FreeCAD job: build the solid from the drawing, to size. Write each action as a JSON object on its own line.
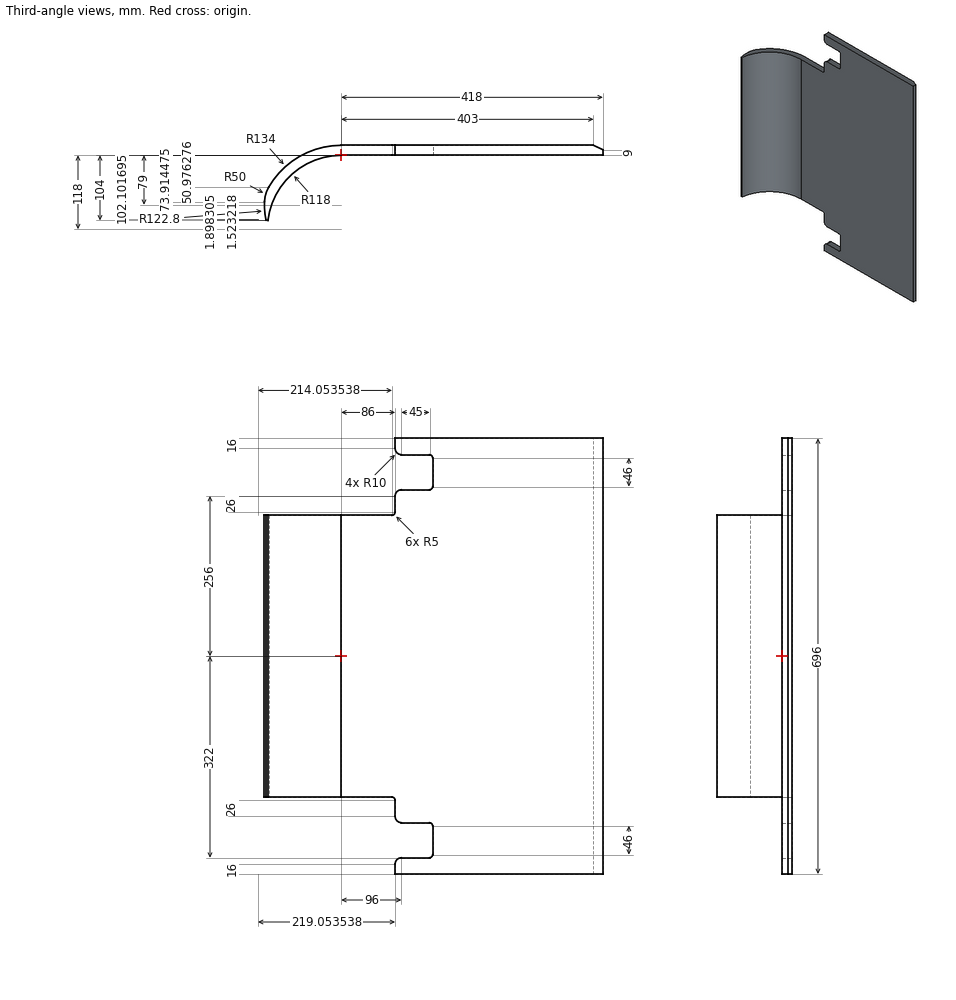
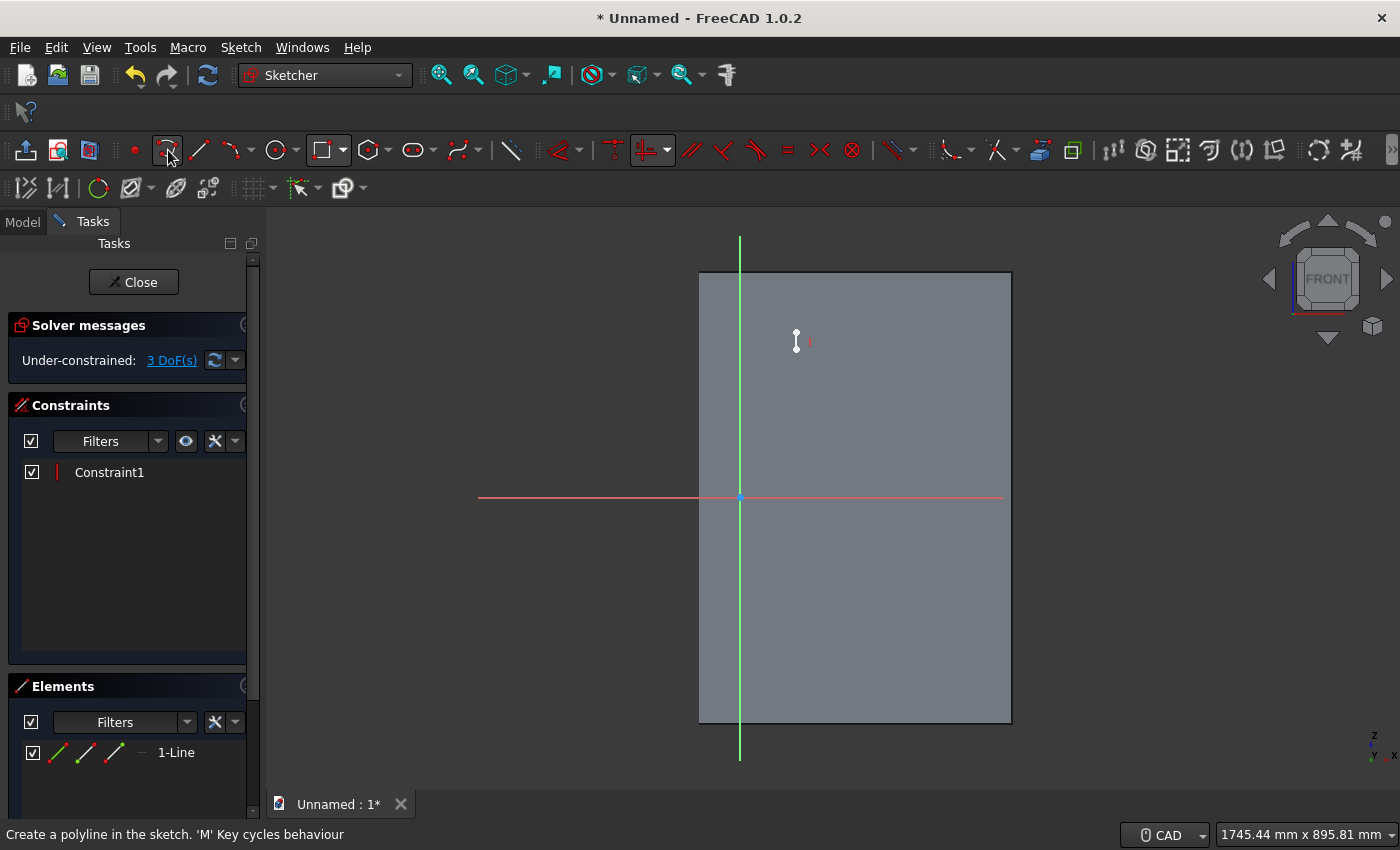
{"action": "scroll", "coordinate": [793, 352], "scroll_direction": "up", "scroll_amount": 7}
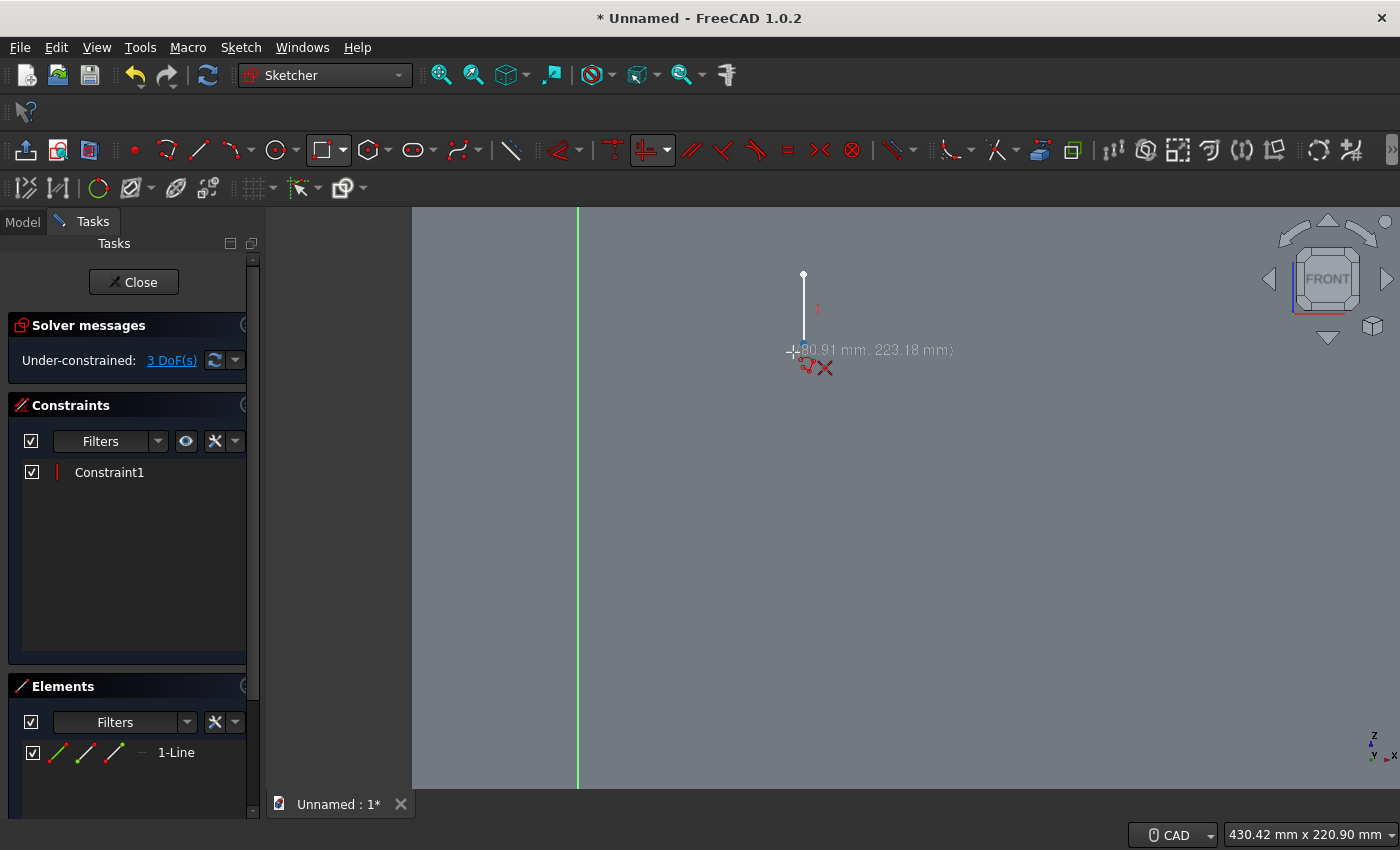
{"action": "left_click", "coordinate": [792, 351]}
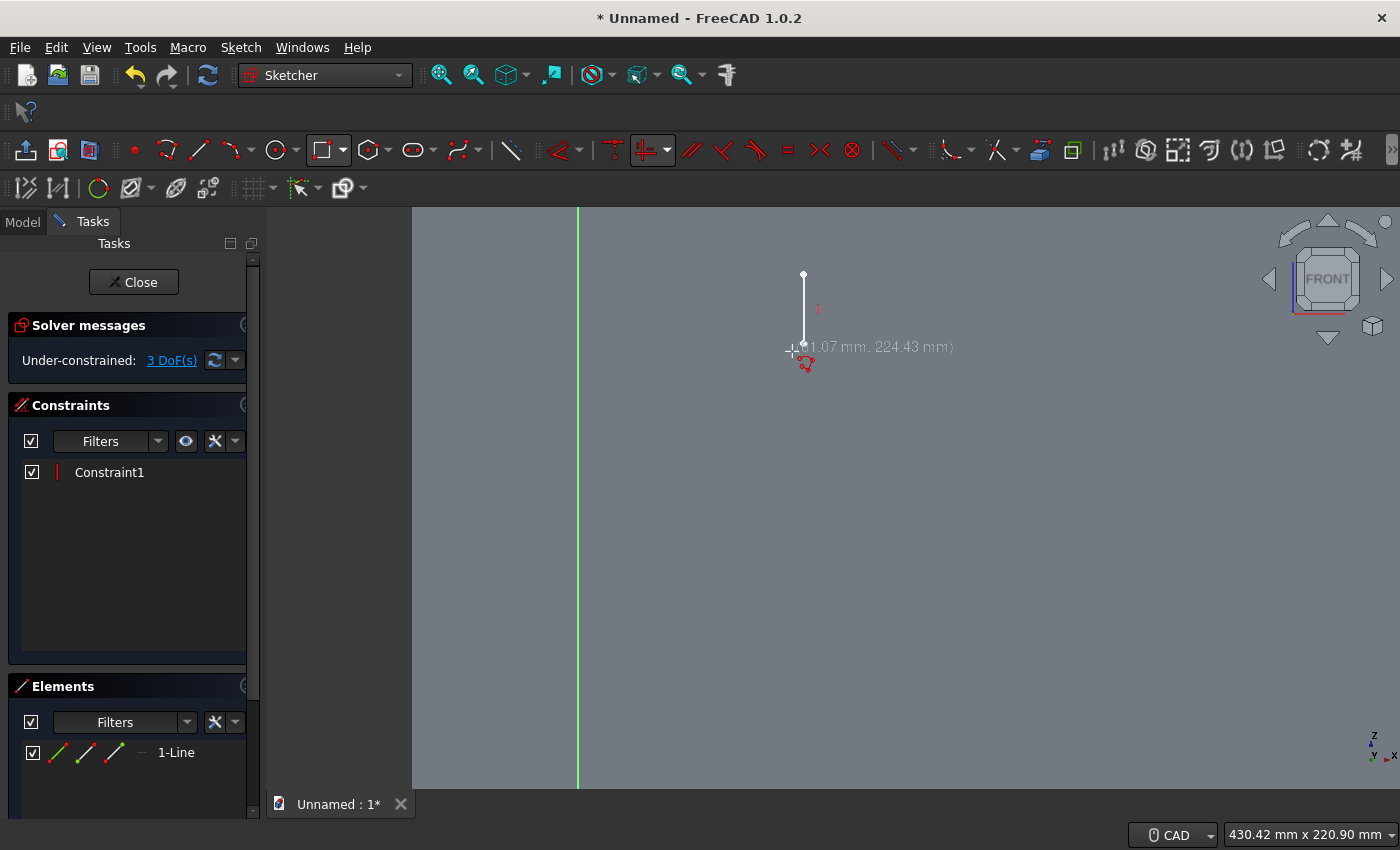
{"action": "scroll", "coordinate": [807, 385], "scroll_direction": "down", "scroll_amount": 8}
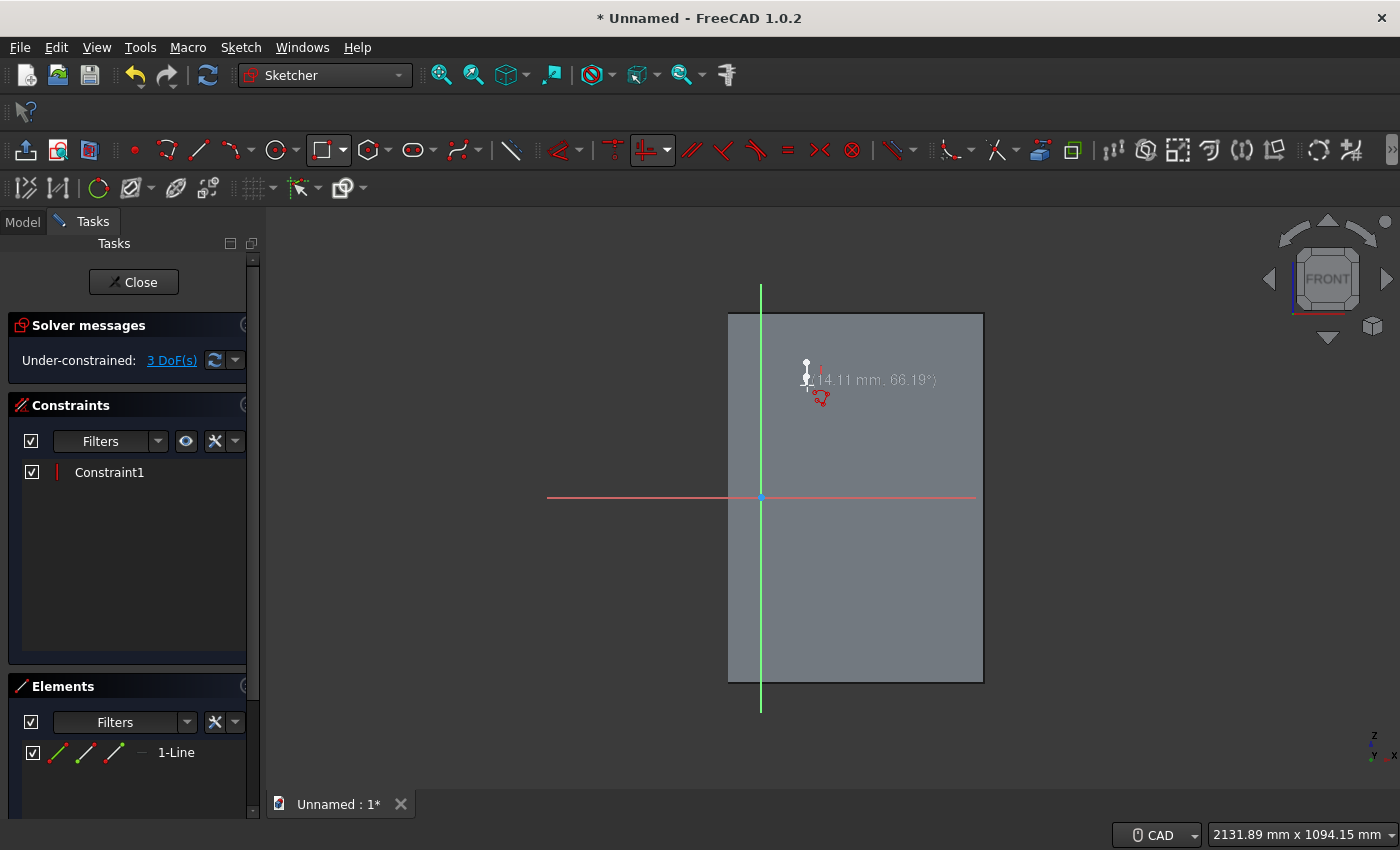
{"action": "left_click", "coordinate": [690, 378]}
{"action": "left_click", "coordinate": [690, 313]}
{"action": "left_click", "coordinate": [807, 313]}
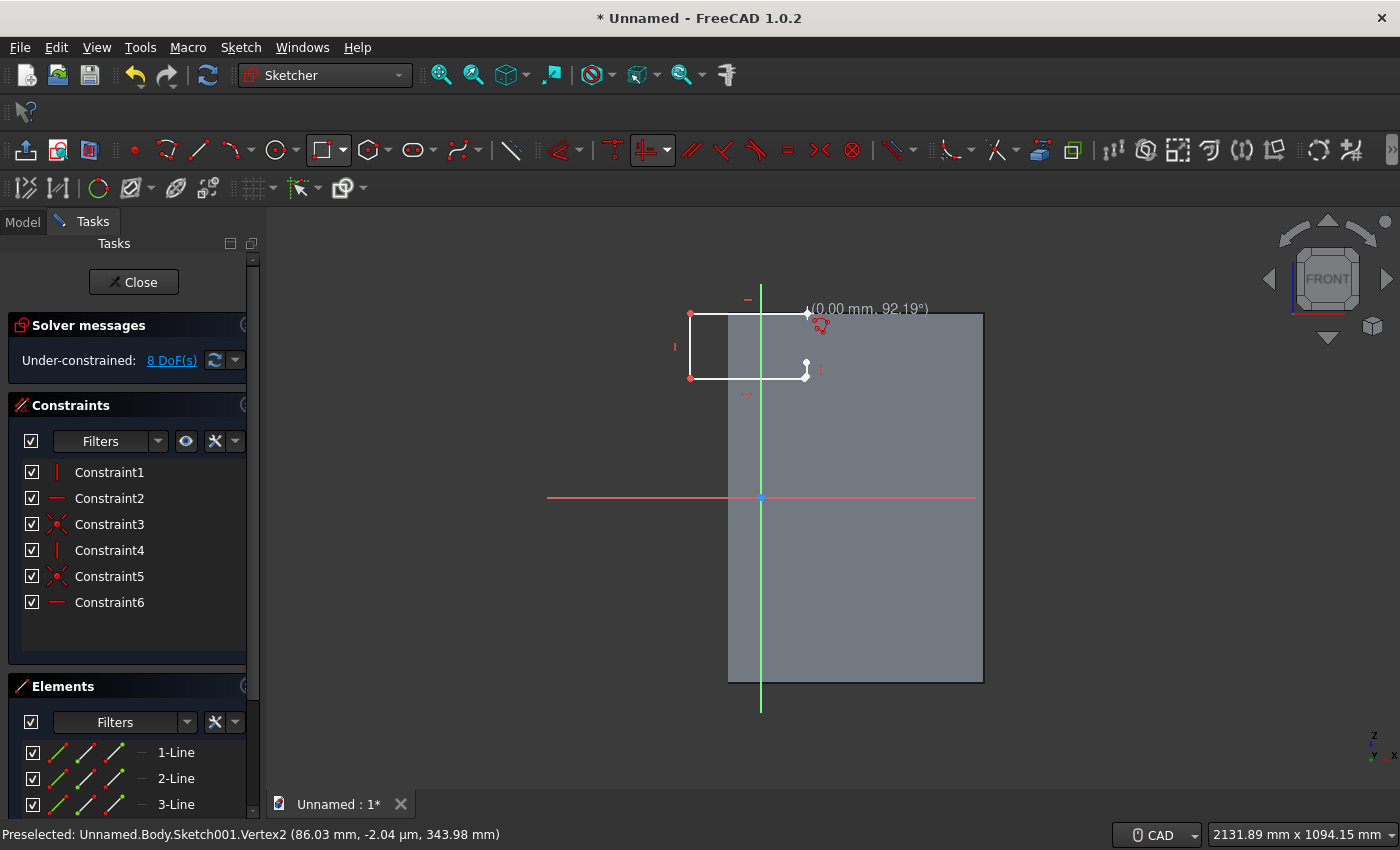
{"action": "scroll", "coordinate": [807, 321], "scroll_direction": "up", "scroll_amount": 4}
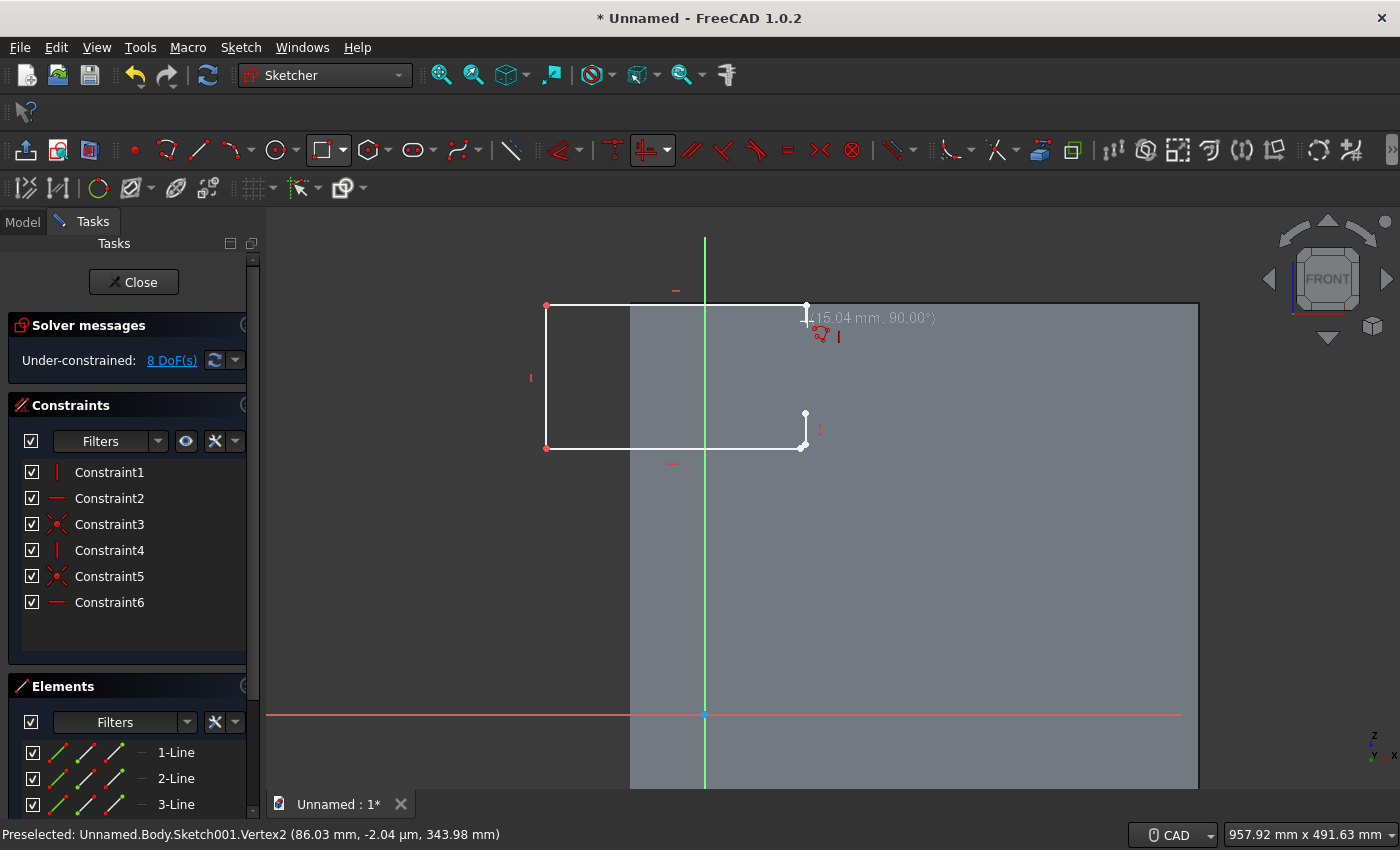
{"action": "left_click", "coordinate": [806, 322]}
{"action": "right_click", "coordinate": [806, 322]}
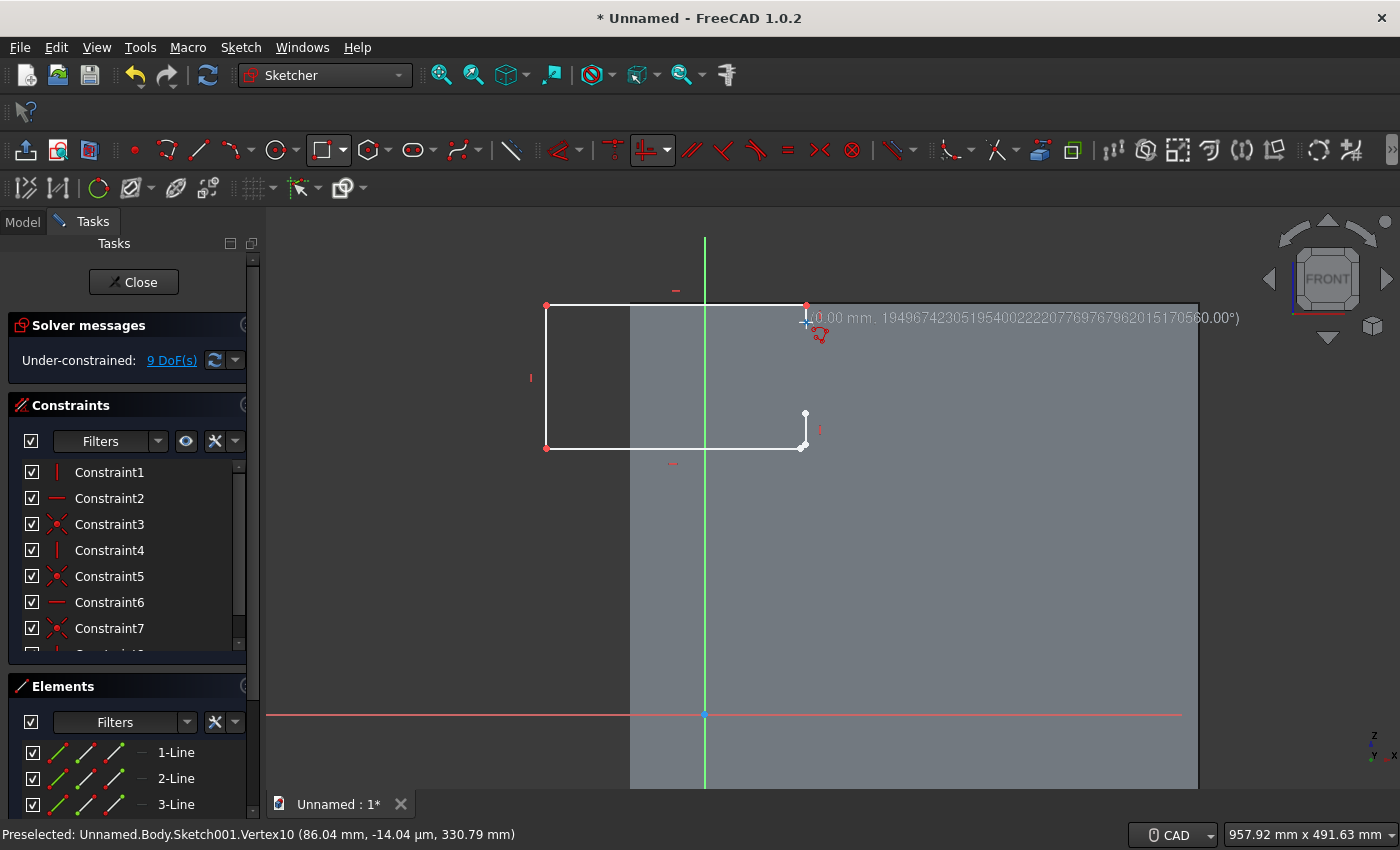
{"action": "left_click", "coordinate": [200, 150]}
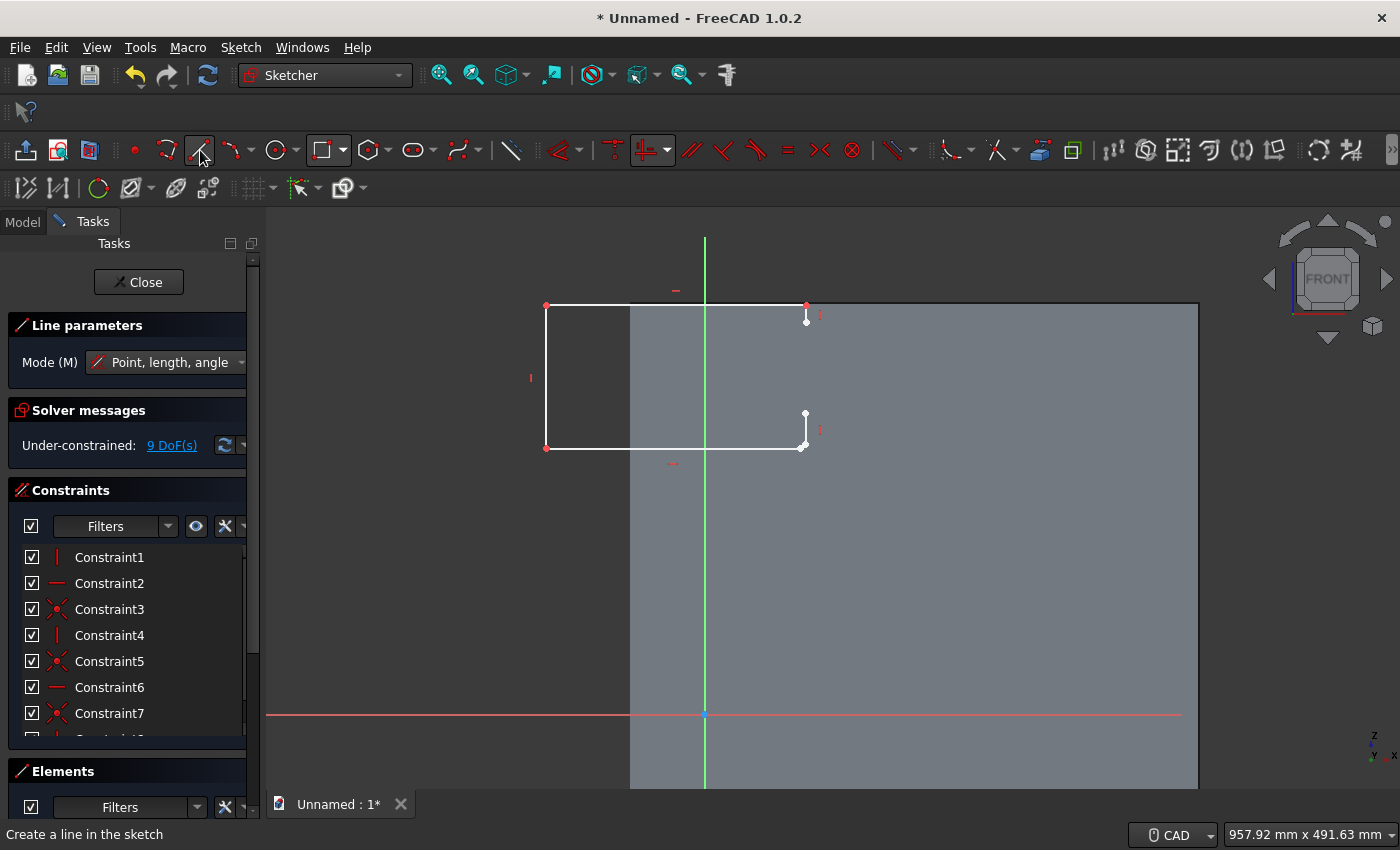
{"action": "left_click", "coordinate": [818, 333]}
{"action": "left_click", "coordinate": [871, 333]}